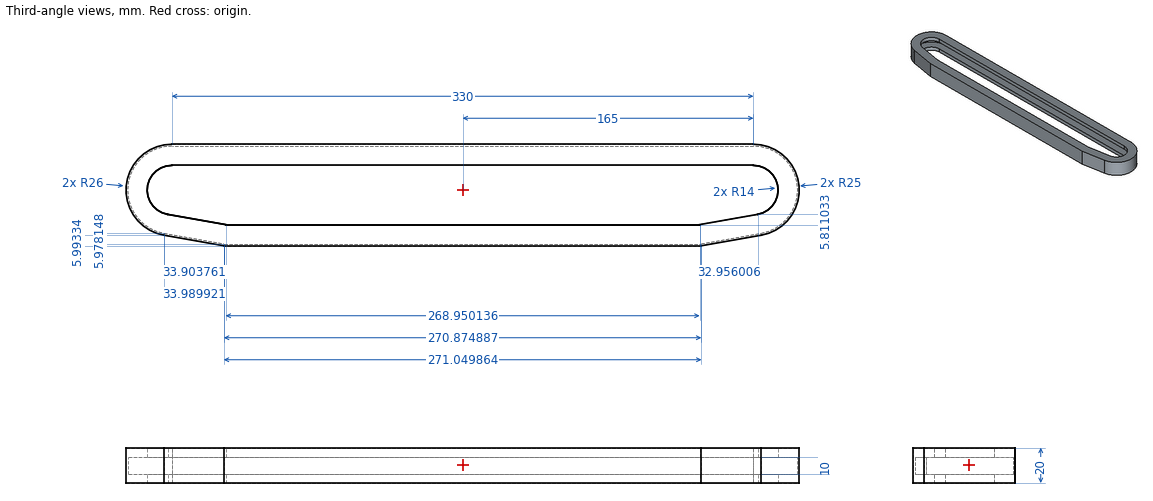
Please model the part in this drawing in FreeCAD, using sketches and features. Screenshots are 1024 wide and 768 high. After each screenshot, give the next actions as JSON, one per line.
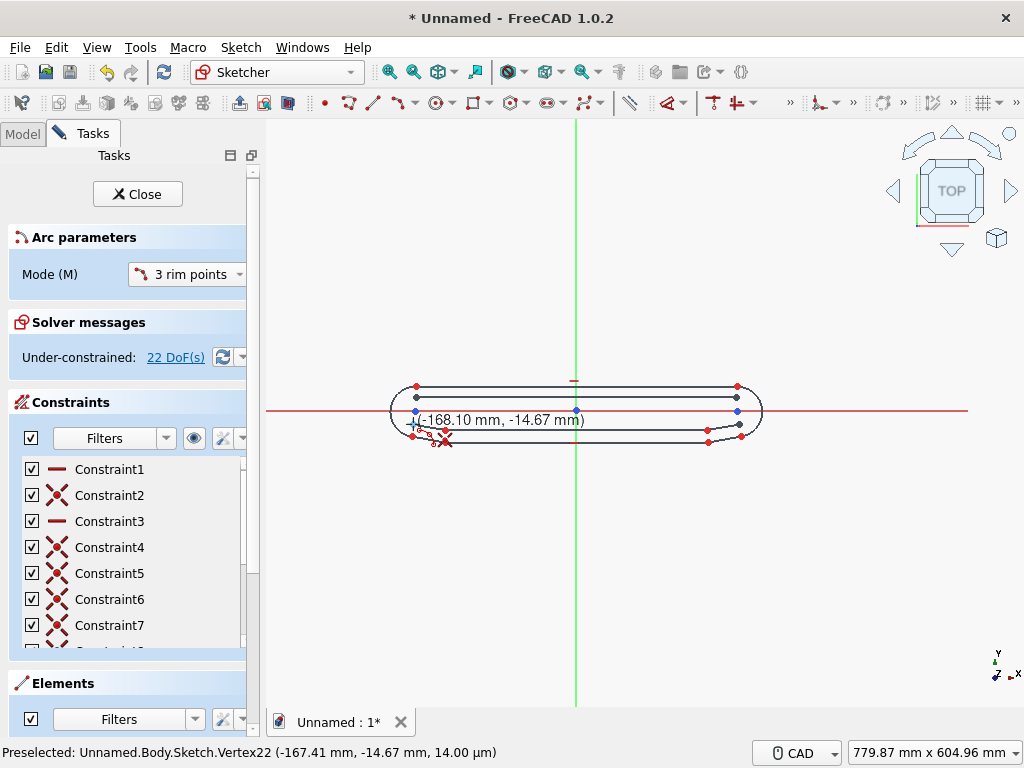
{"action": "scroll", "coordinate": [737, 397], "scroll_direction": "up", "scroll_amount": 2}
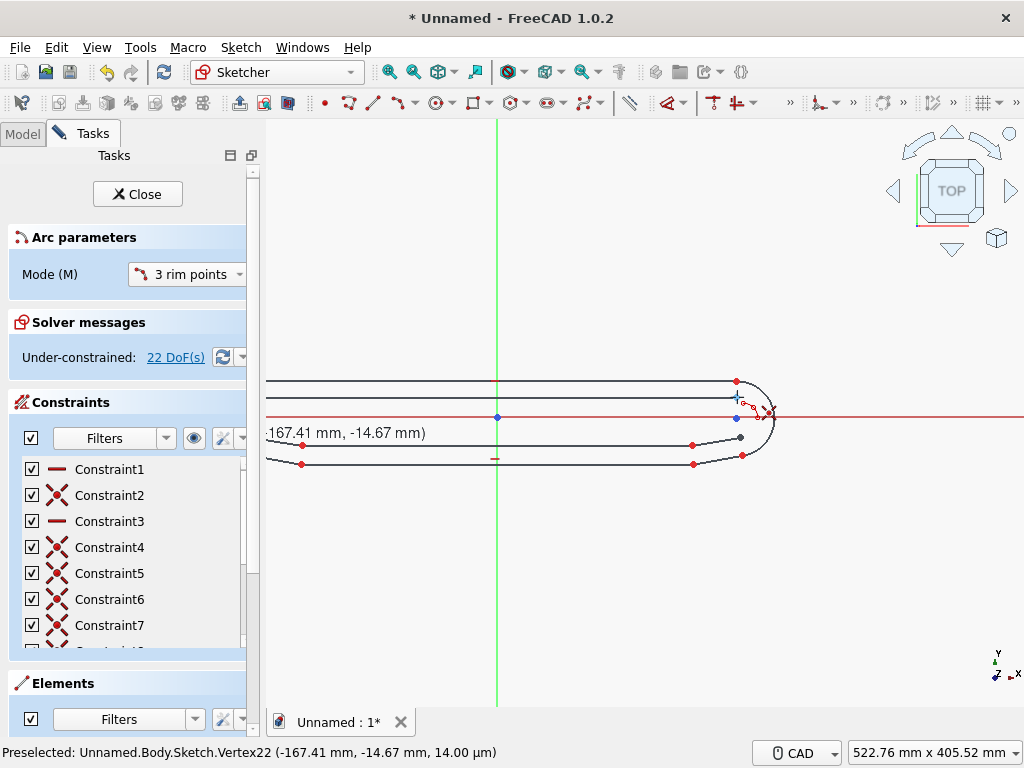
{"action": "left_click", "coordinate": [736, 398]}
{"action": "left_click", "coordinate": [740, 438]}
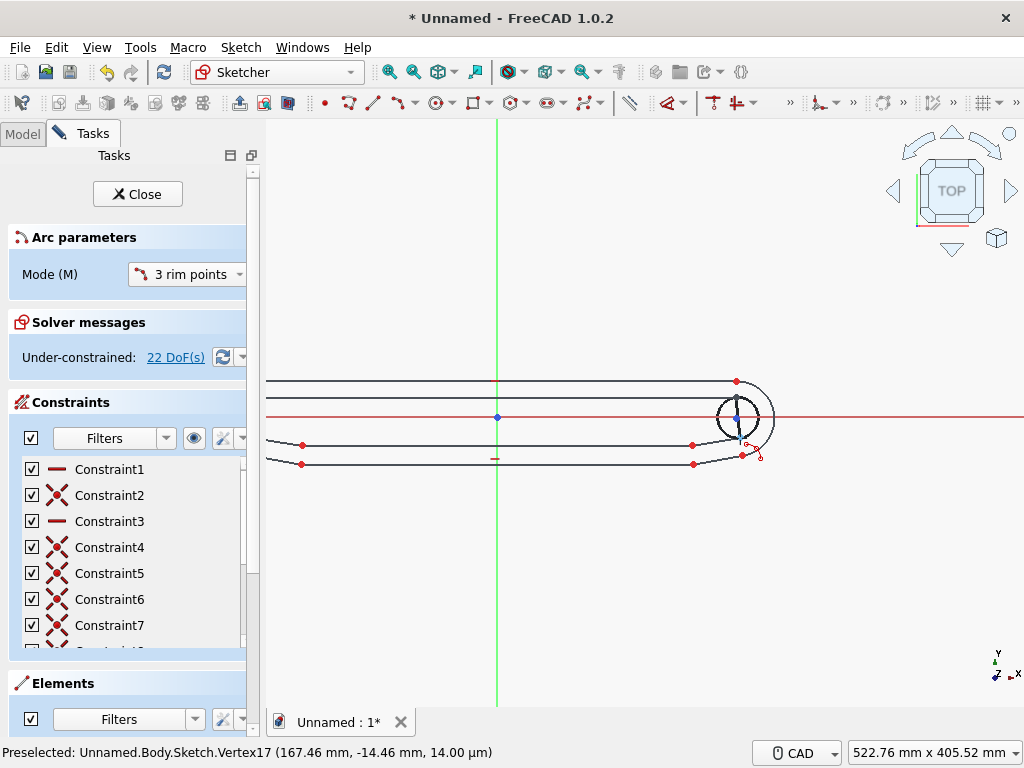
{"action": "scroll", "coordinate": [752, 404], "scroll_direction": "up", "scroll_amount": 2}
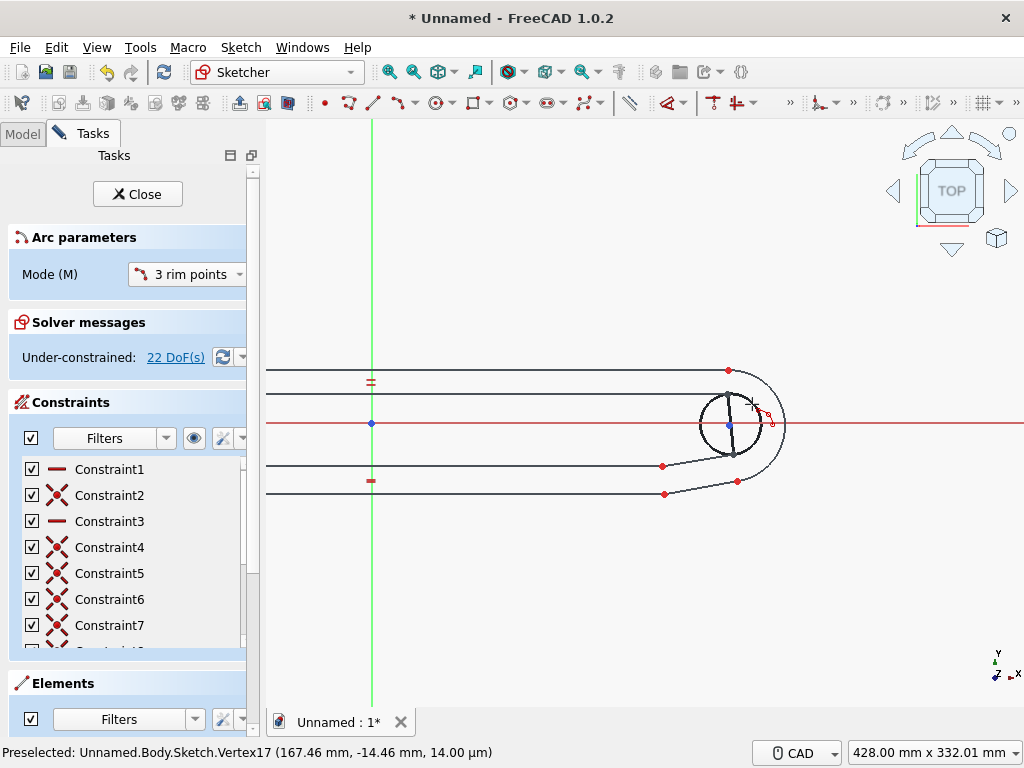
{"action": "left_click", "coordinate": [752, 404]}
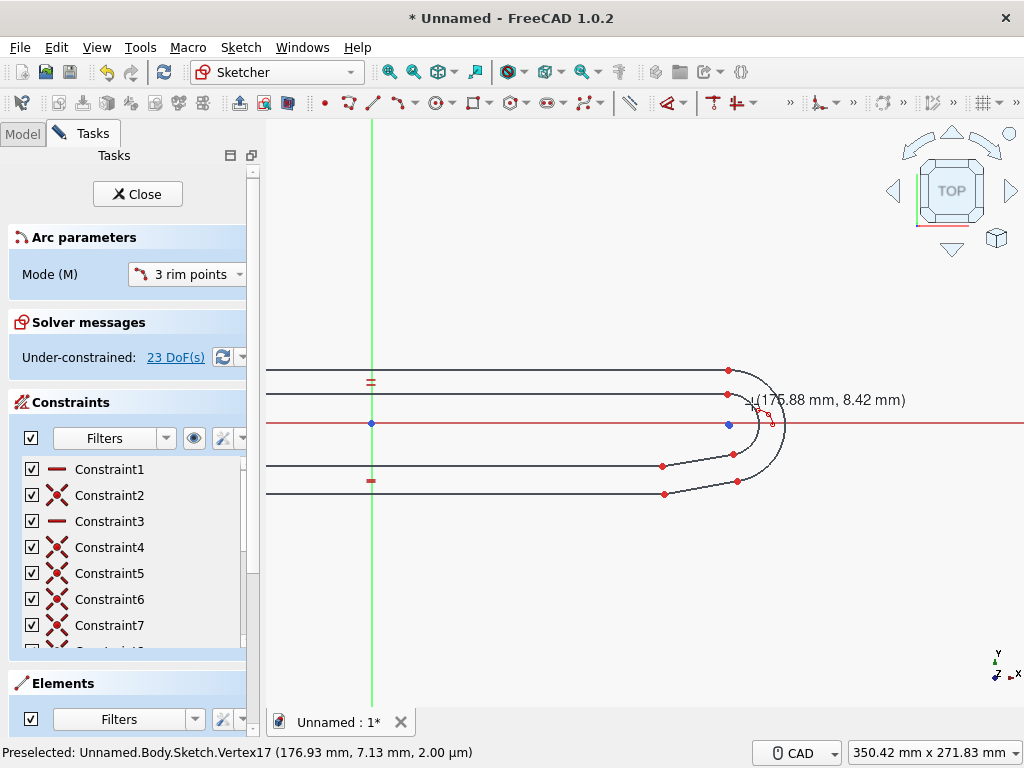
{"action": "scroll", "coordinate": [744, 400], "scroll_direction": "down", "scroll_amount": 4}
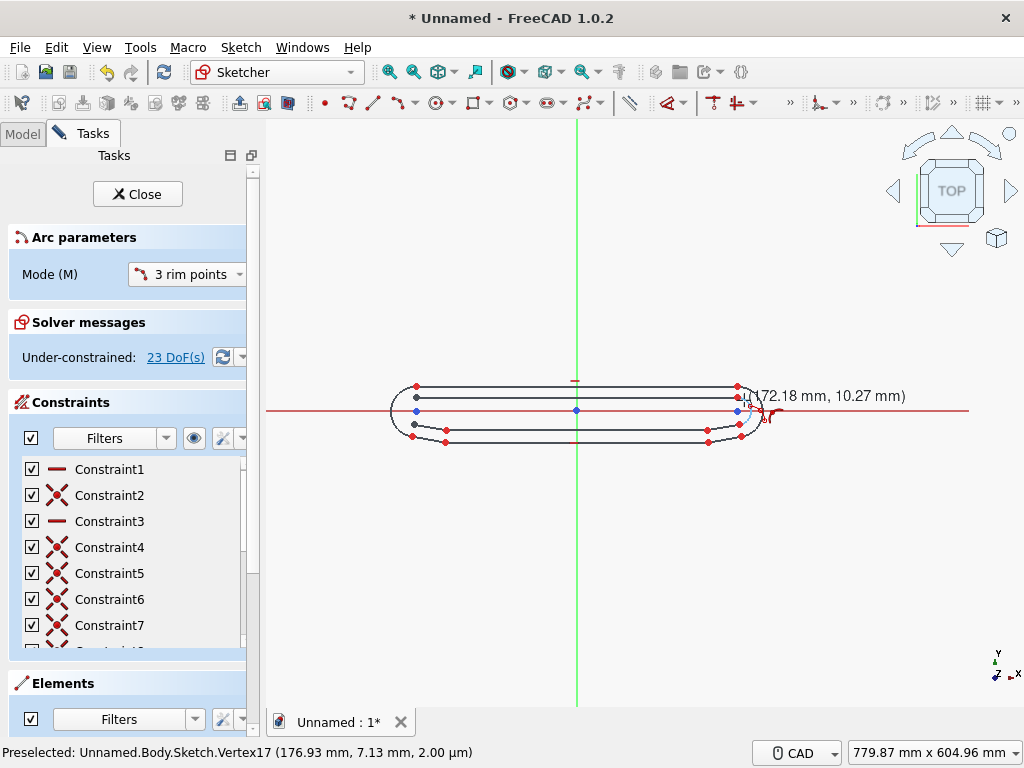
{"action": "scroll", "coordinate": [414, 424], "scroll_direction": "up", "scroll_amount": 2}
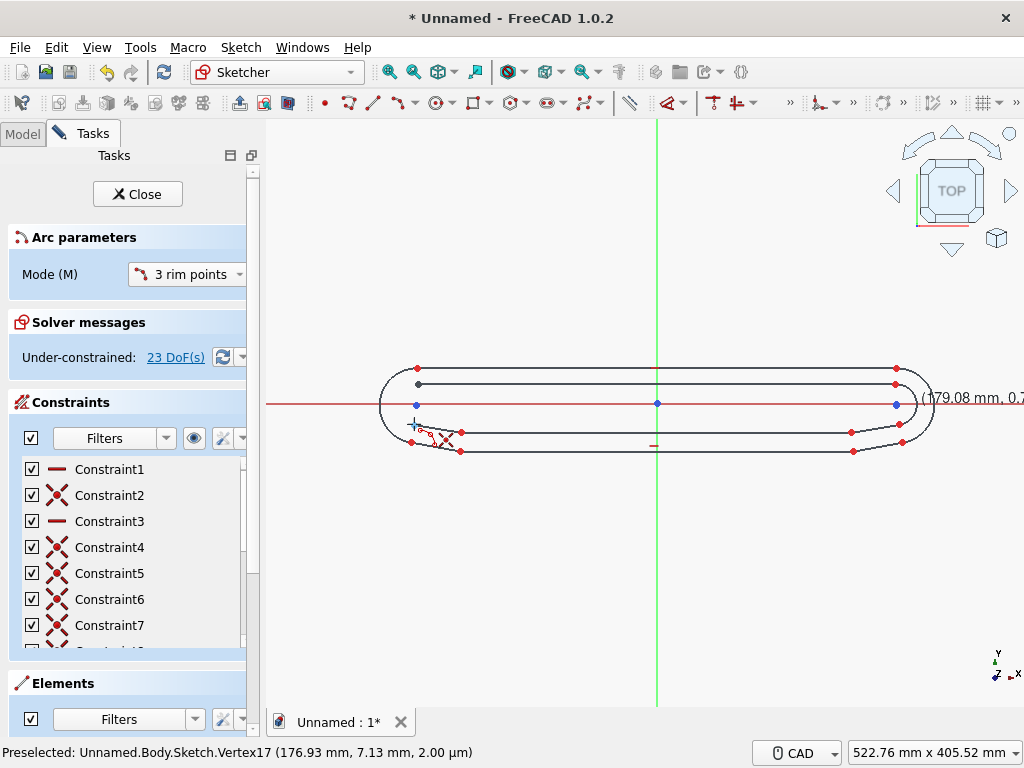
{"action": "left_click", "coordinate": [414, 425]}
{"action": "left_click", "coordinate": [418, 384]}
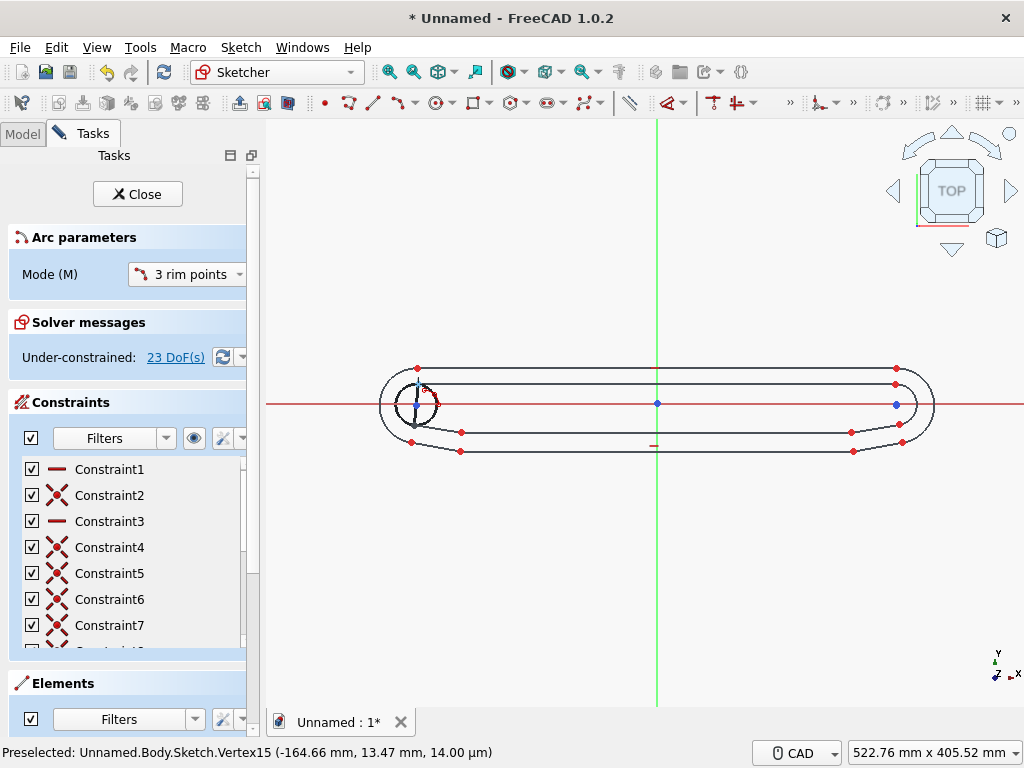
{"action": "scroll", "coordinate": [402, 391], "scroll_direction": "up", "scroll_amount": 2}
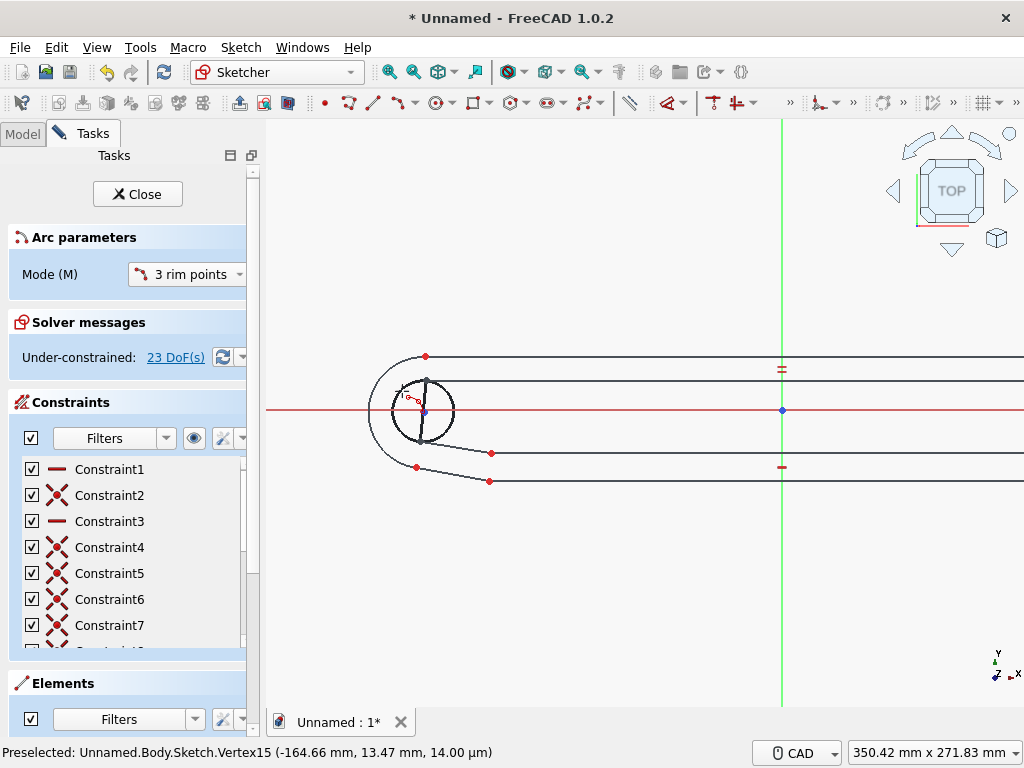
{"action": "left_click", "coordinate": [402, 391]}
{"action": "key", "text": "Escape"}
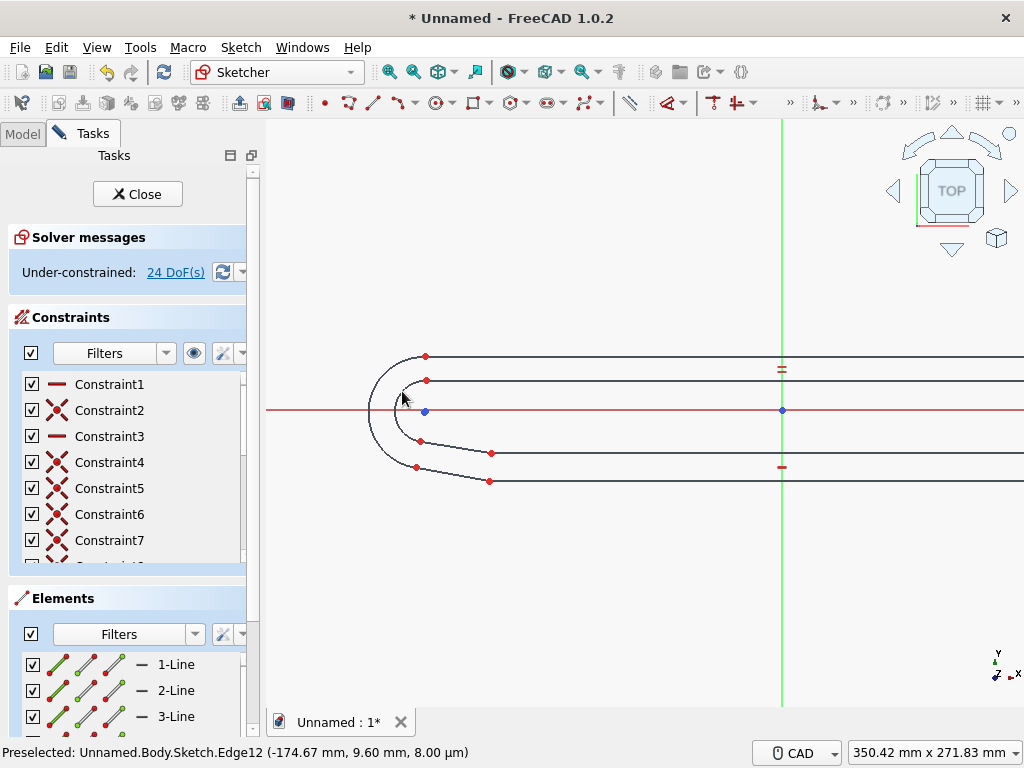
{"action": "left_click", "coordinate": [640, 357]}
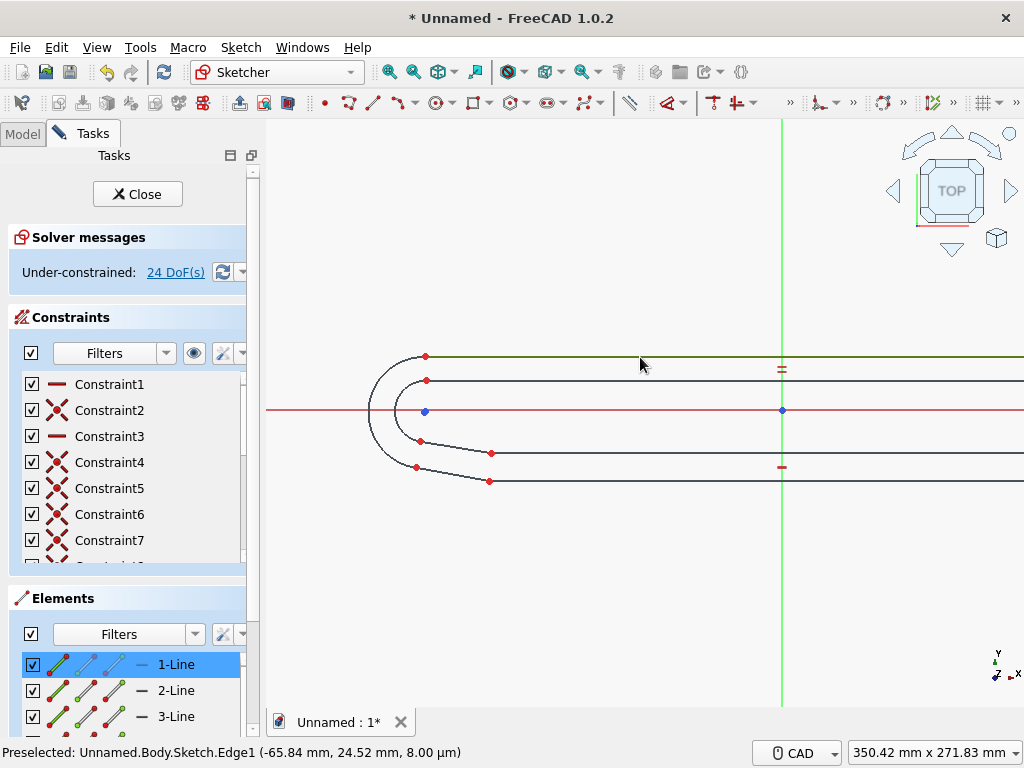
{"action": "left_click", "coordinate": [381, 377]}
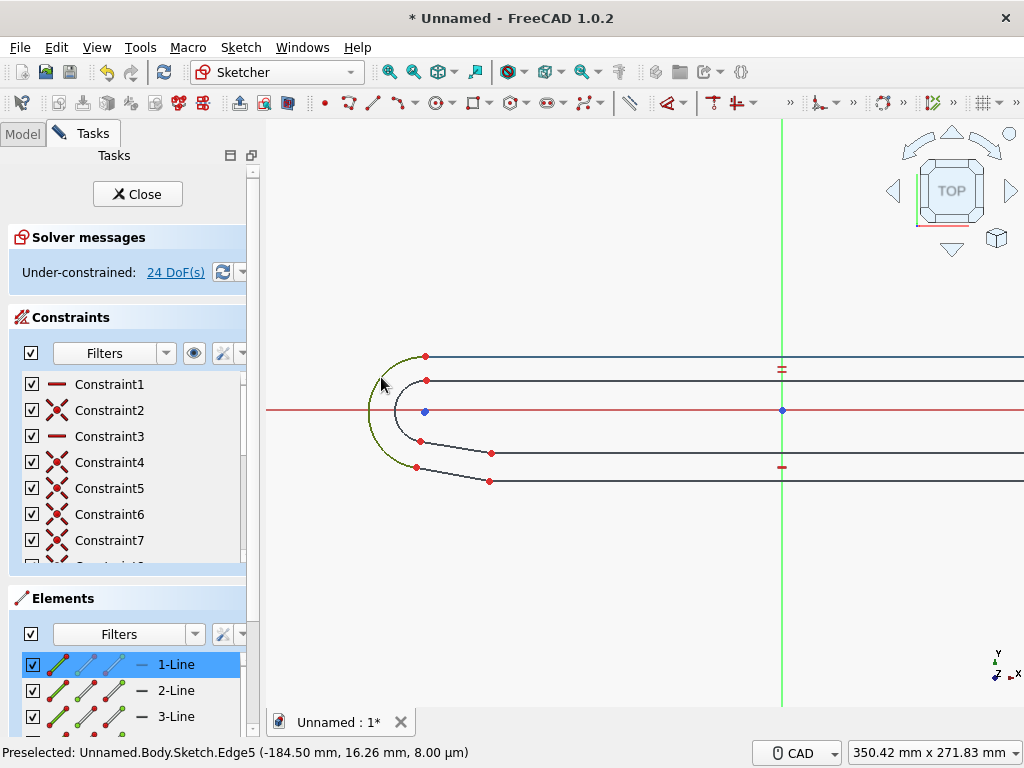
{"action": "key", "text": "t"}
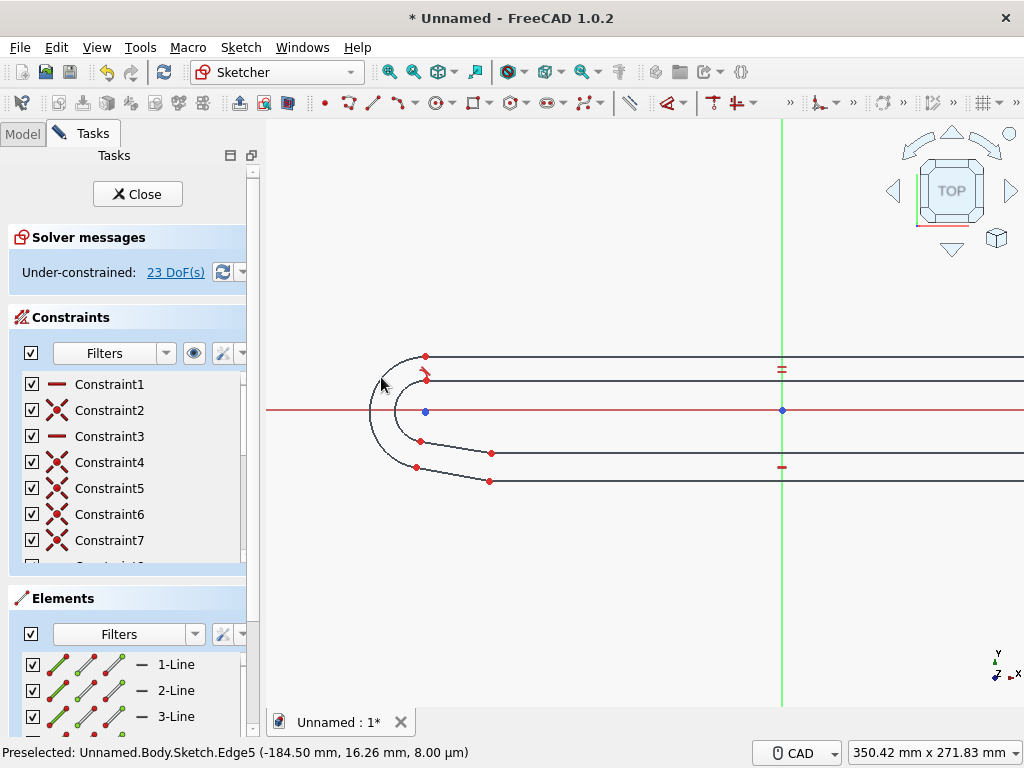
{"action": "left_click", "coordinate": [640, 357]}